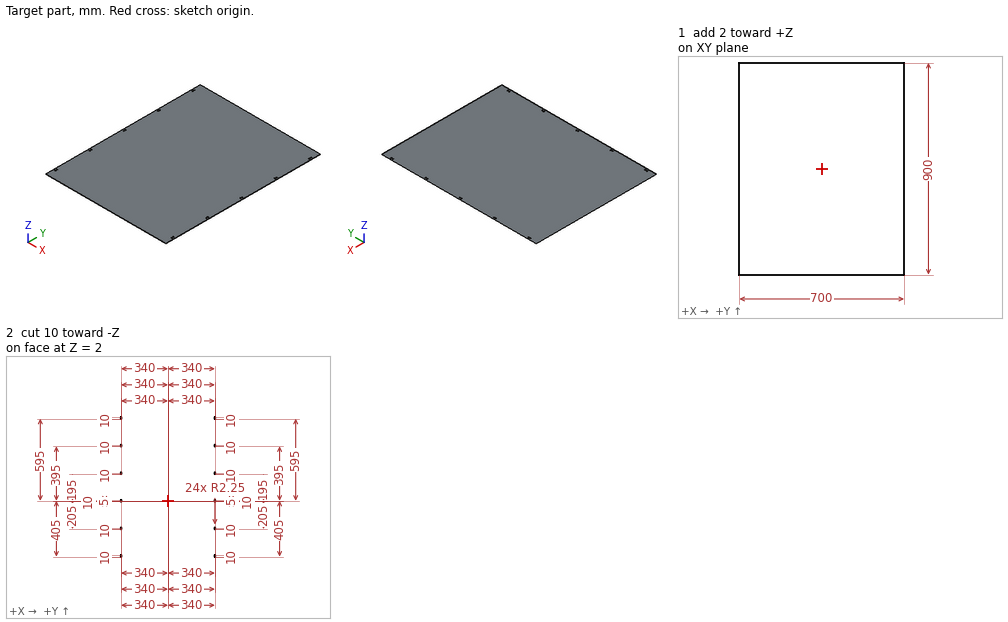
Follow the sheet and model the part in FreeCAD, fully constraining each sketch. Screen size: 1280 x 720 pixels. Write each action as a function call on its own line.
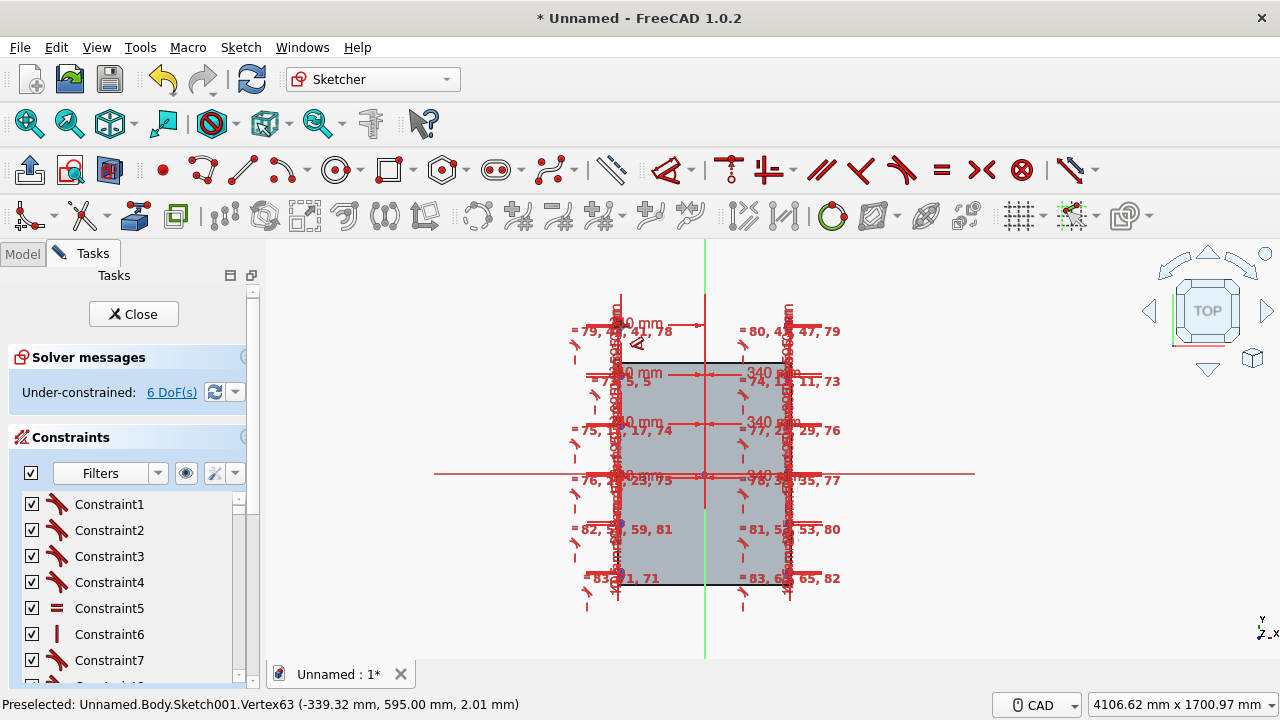
scroll(789, 327, up, 14)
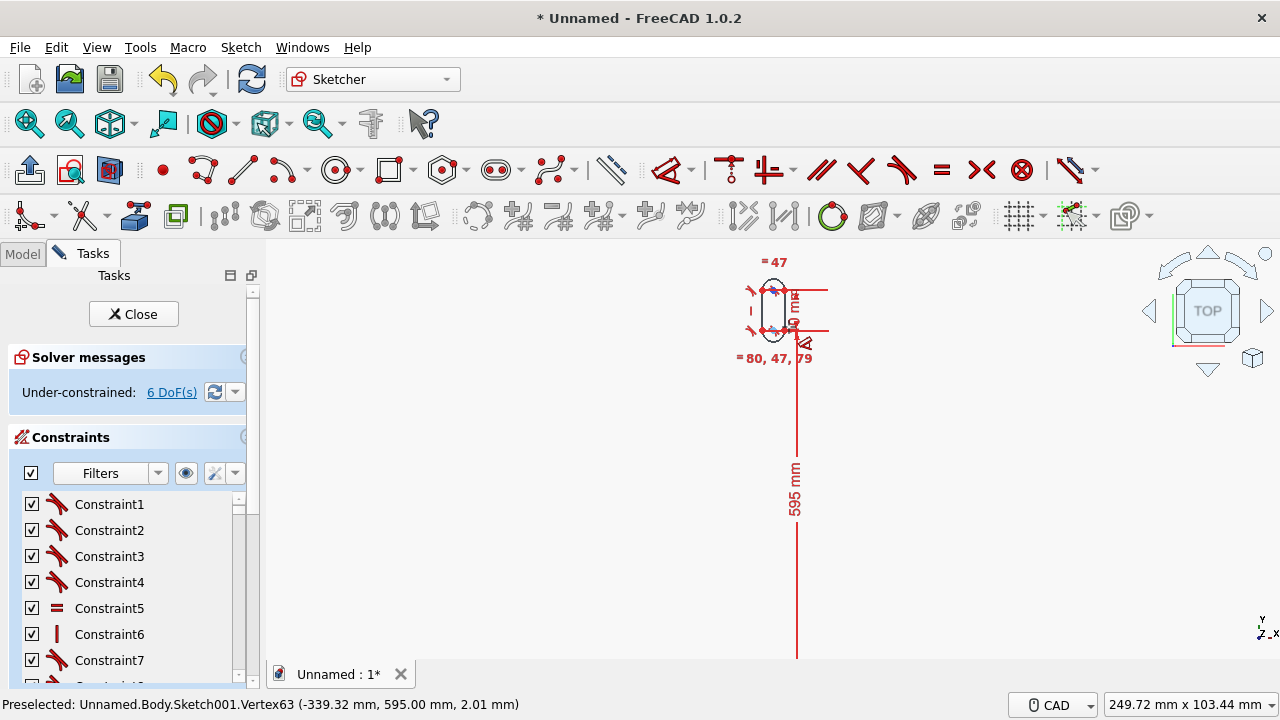
click(774, 331)
click(534, 297)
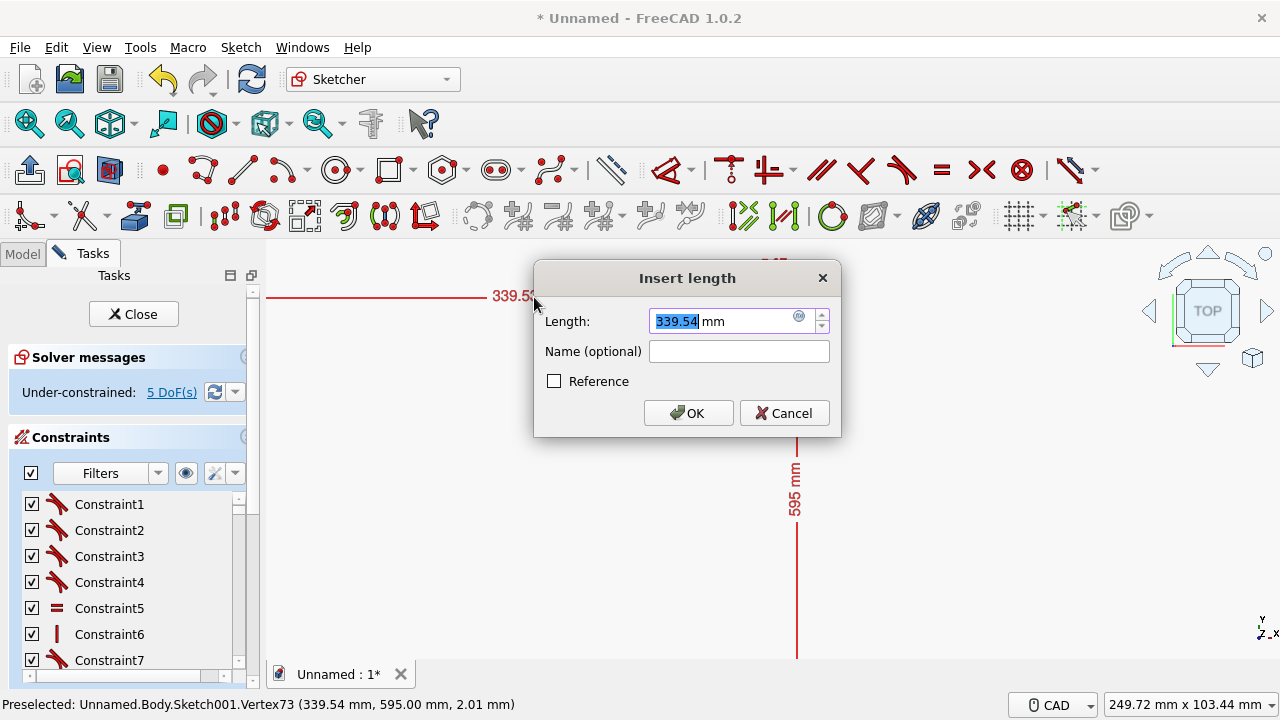
text(340)
key(Return)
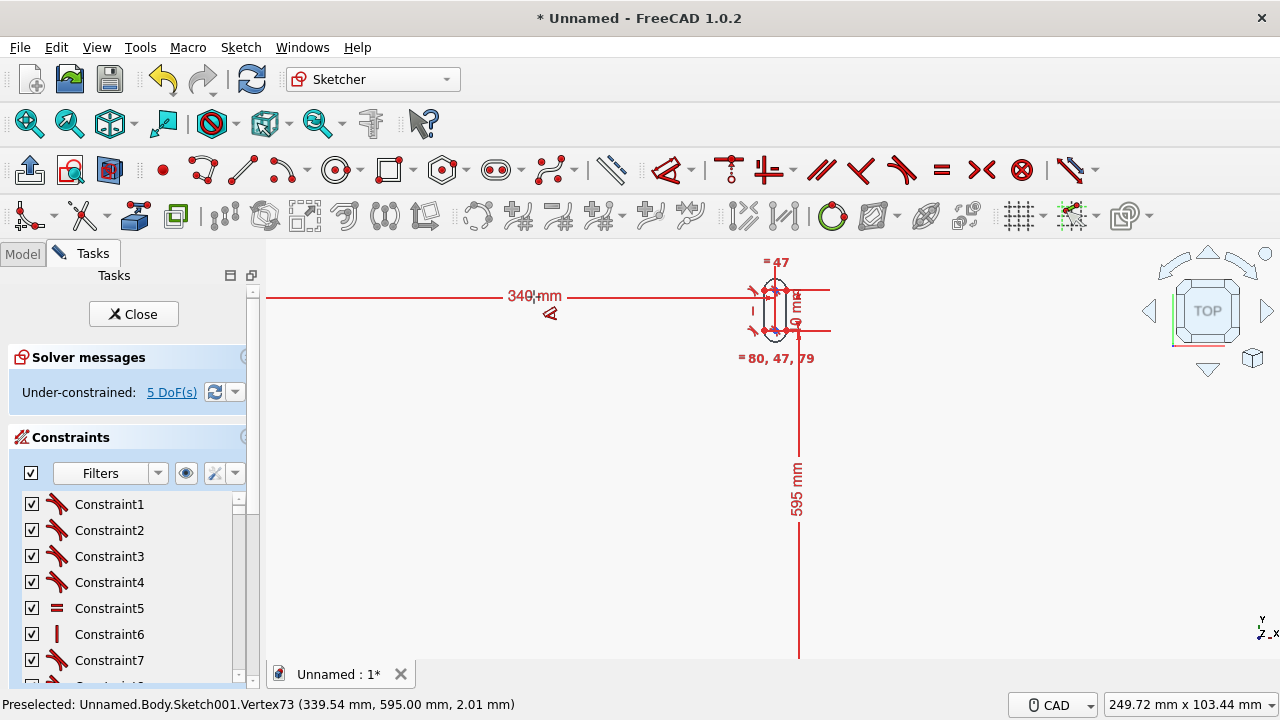
scroll(789, 327, down, 14)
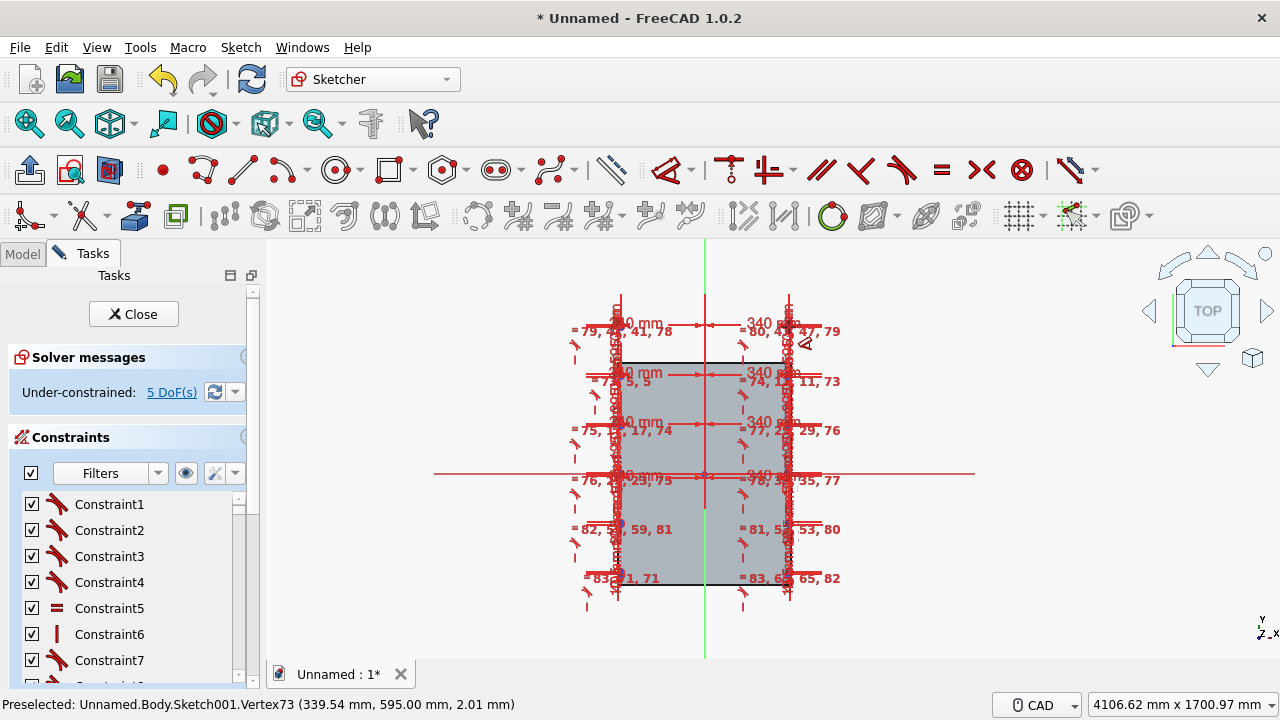
scroll(789, 525, up, 14)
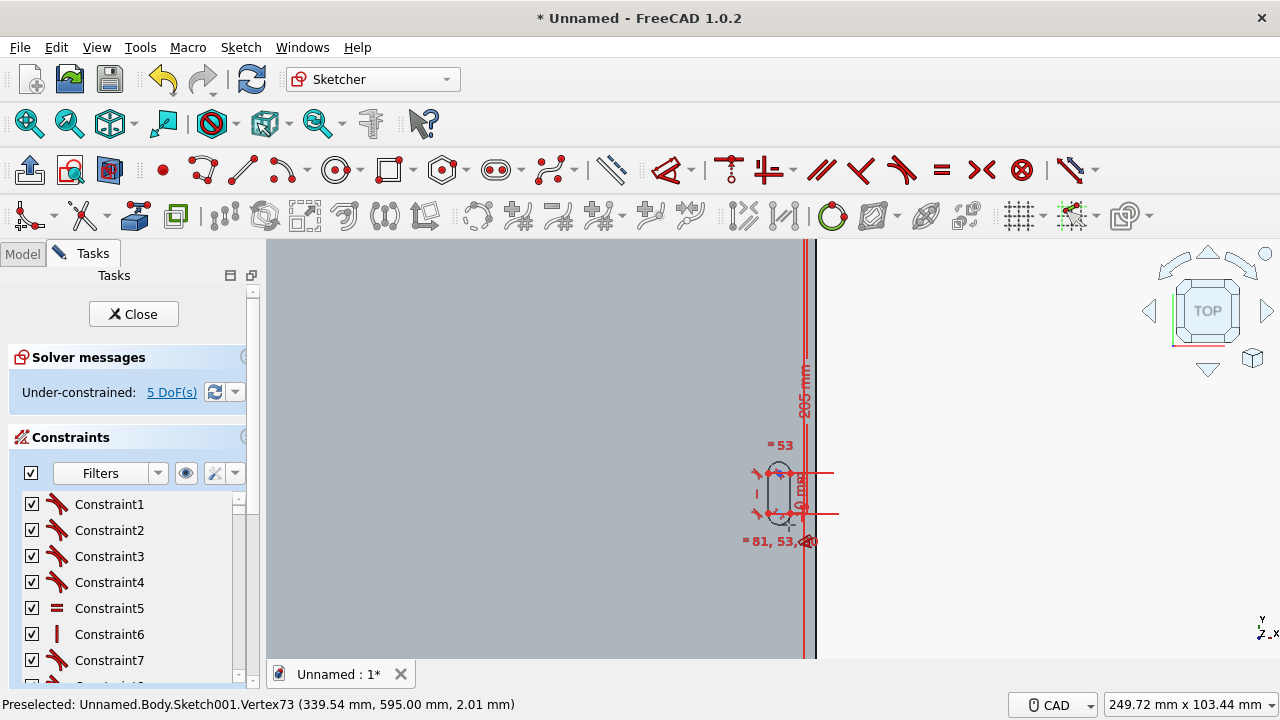
click(779, 514)
click(537, 548)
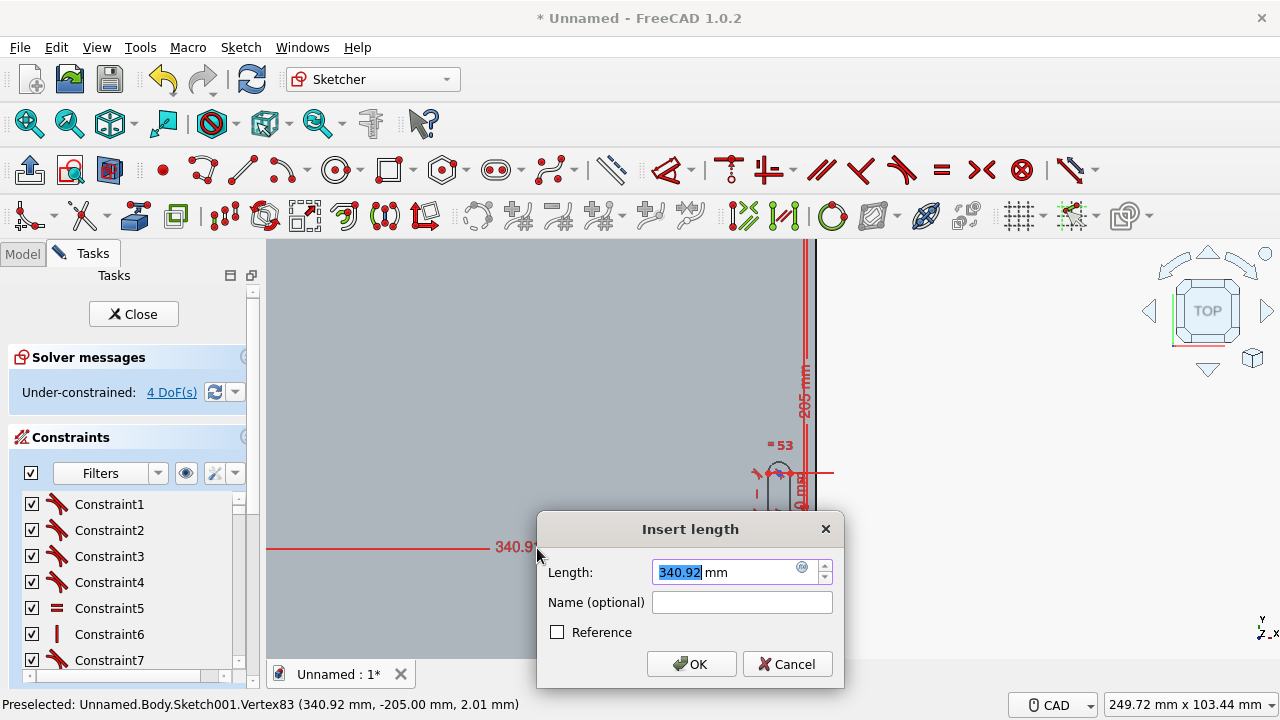
text(340)
key(Return)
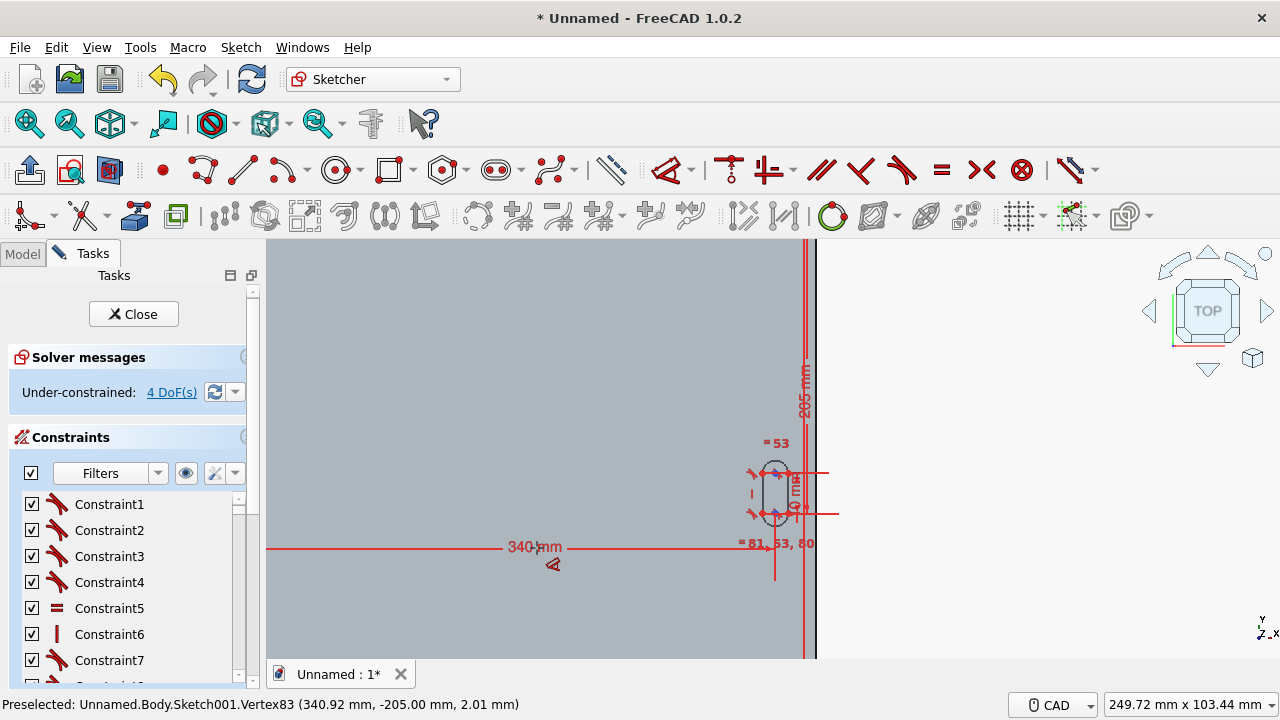
scroll(789, 525, down, 14)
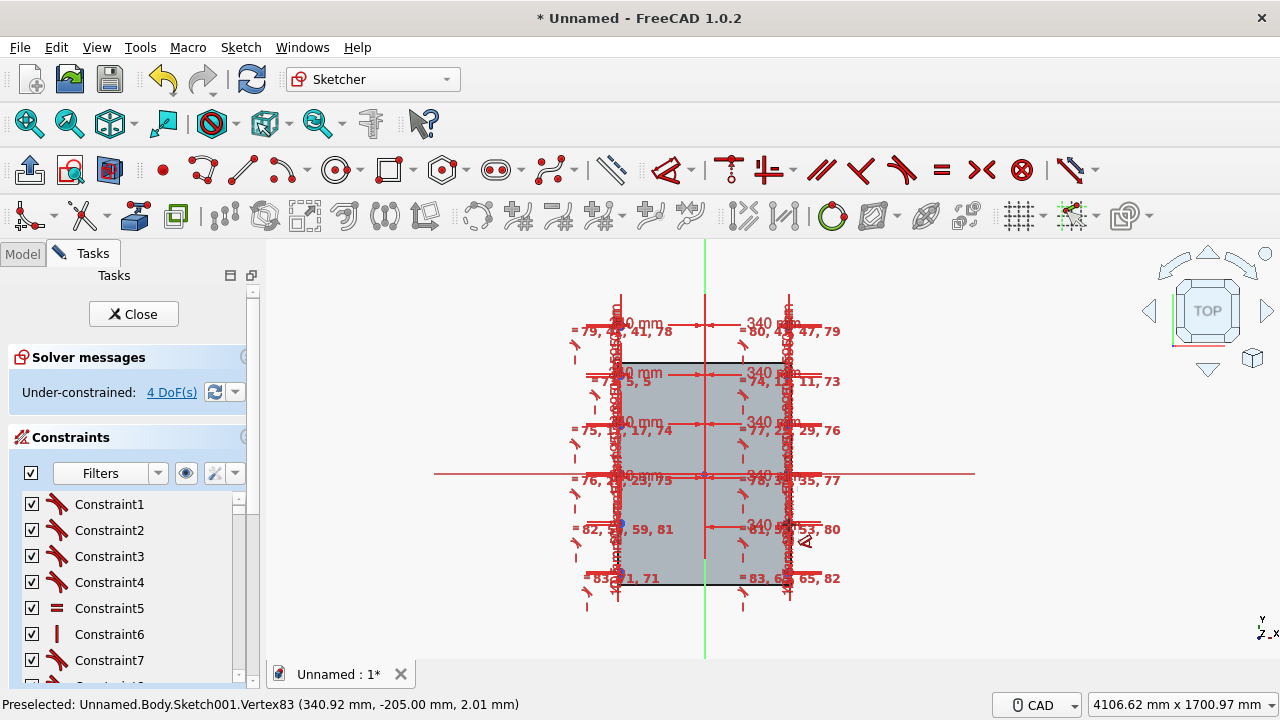
scroll(621, 525, up, 14)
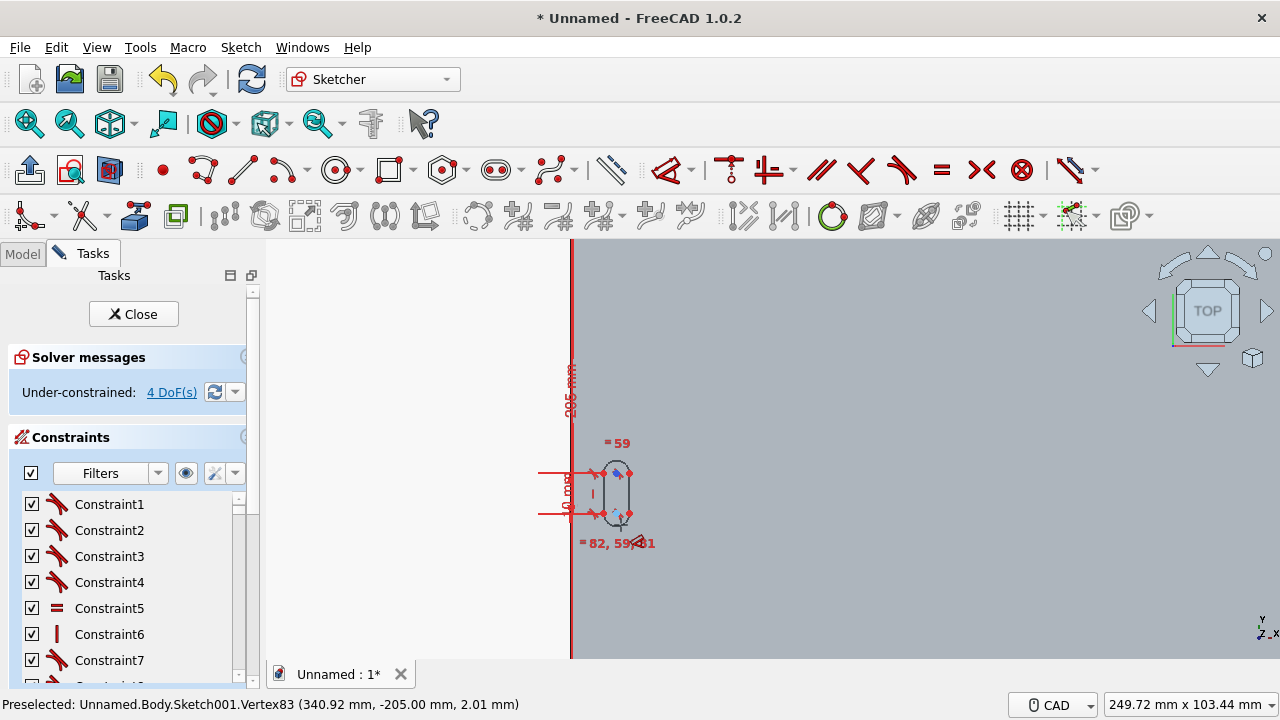
click(617, 514)
click(866, 548)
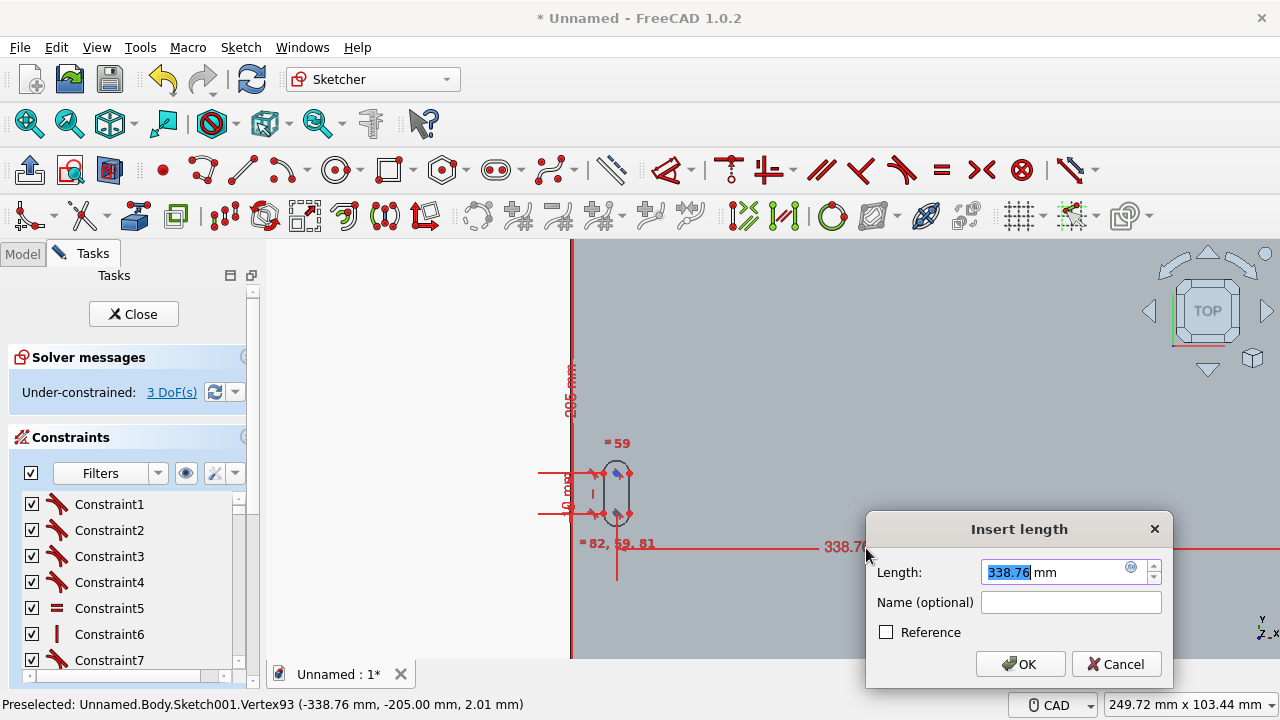
text(340)
key(Return)